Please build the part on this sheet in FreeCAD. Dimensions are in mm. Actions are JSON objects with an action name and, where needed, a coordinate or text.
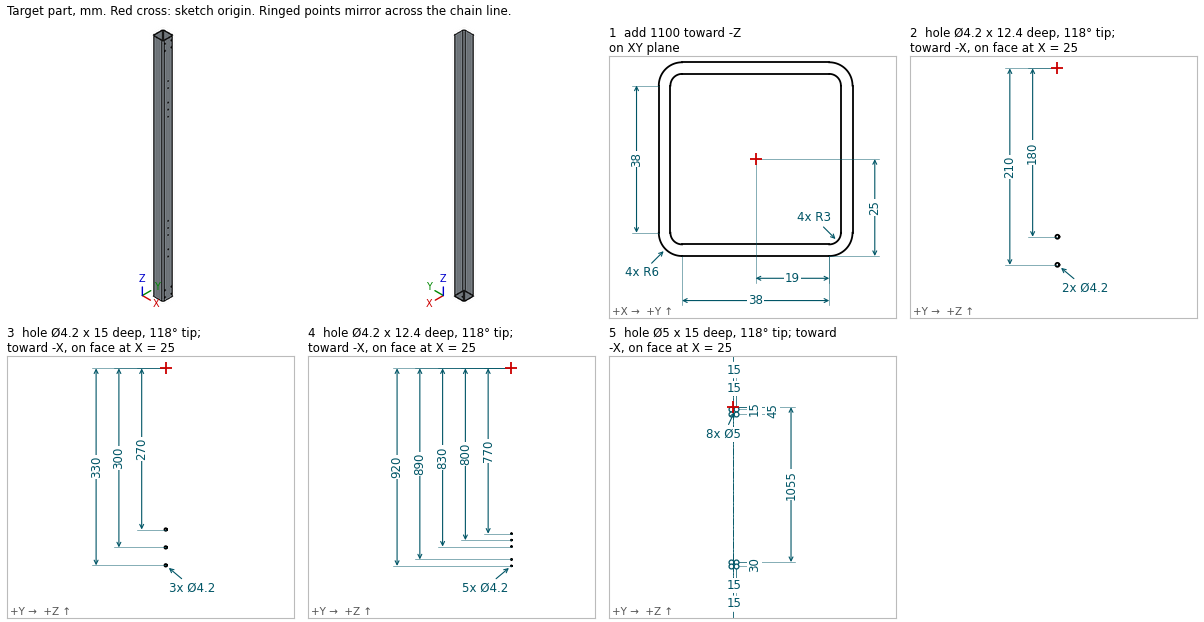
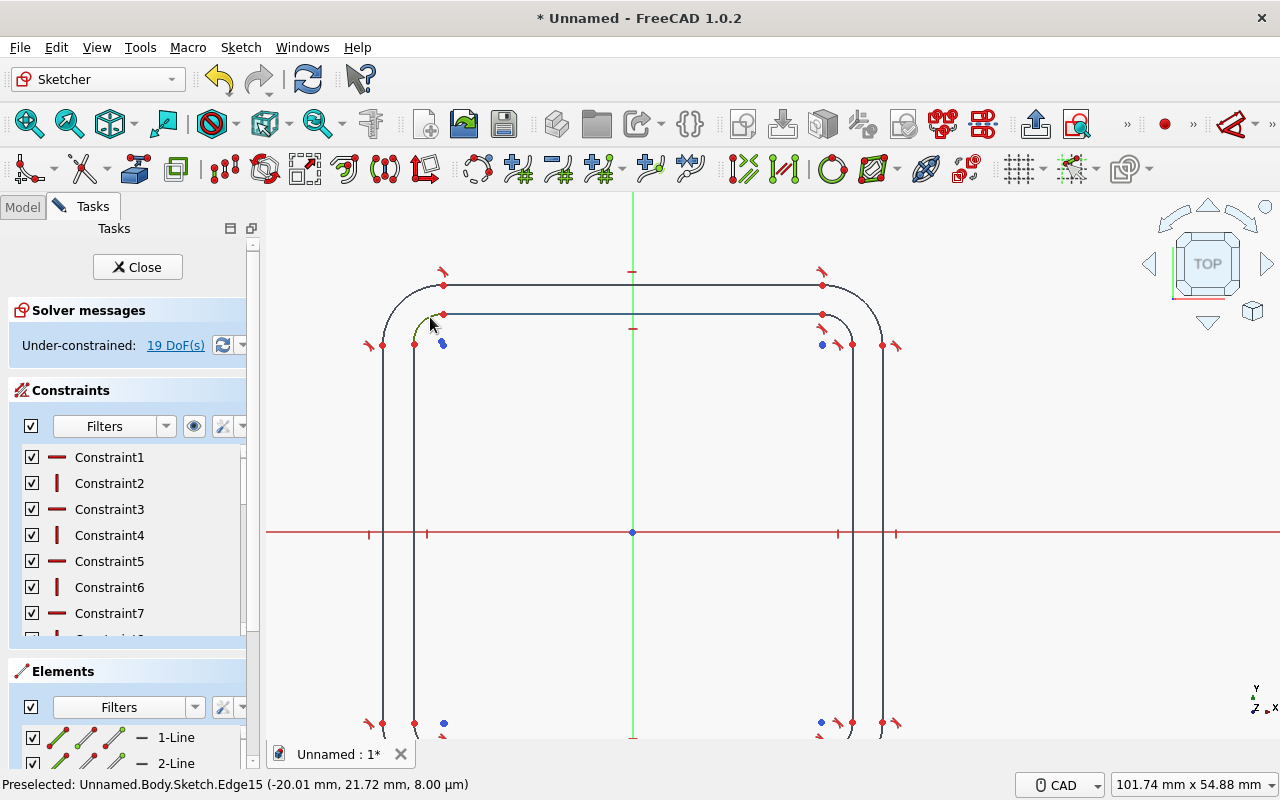
{"action": "key", "text": "t"}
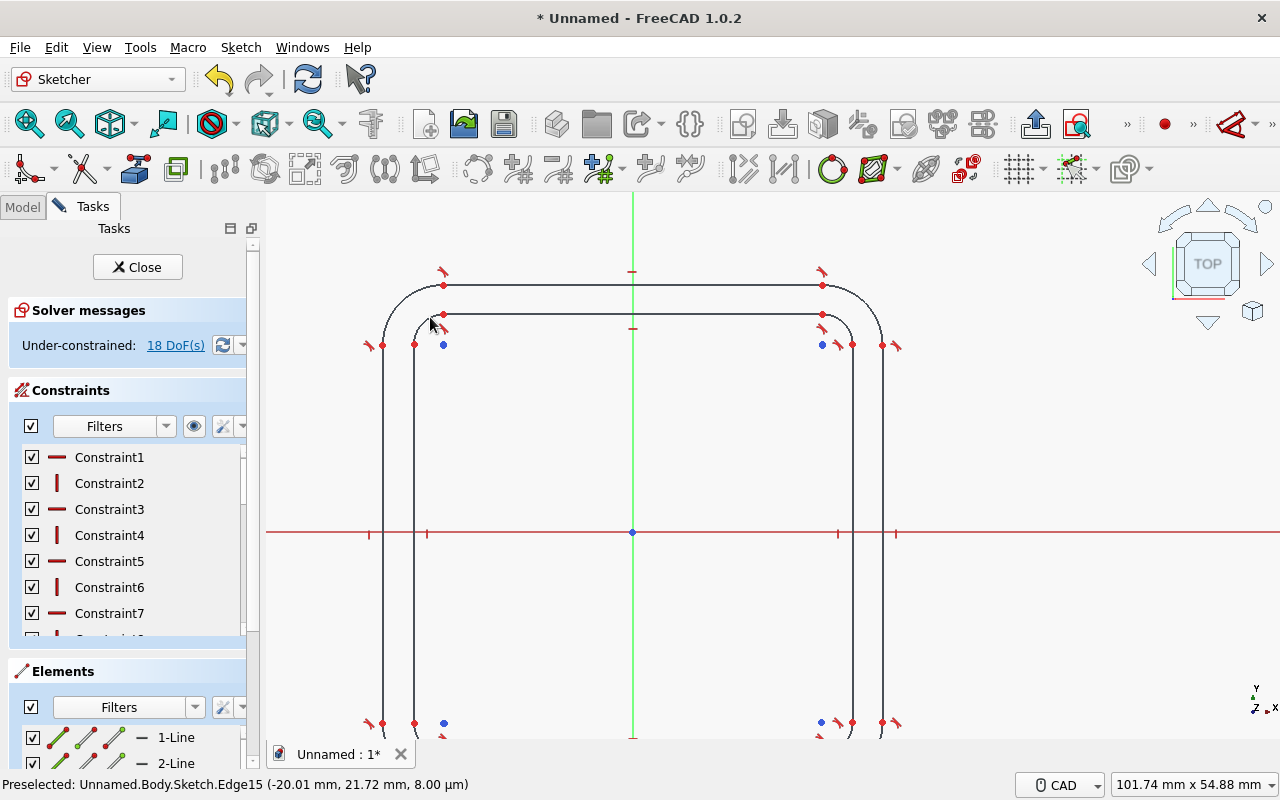
{"action": "left_click", "coordinate": [414, 458]}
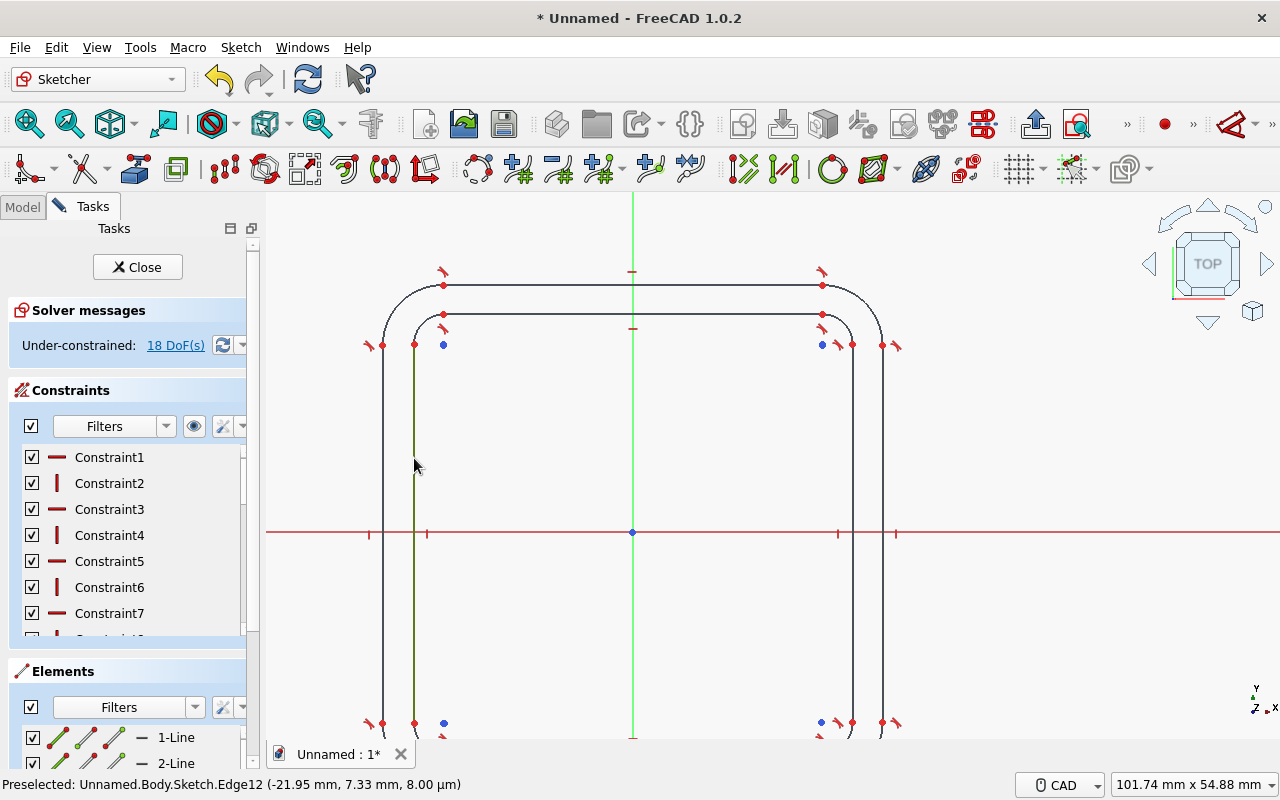
{"action": "left_click", "coordinate": [430, 318]}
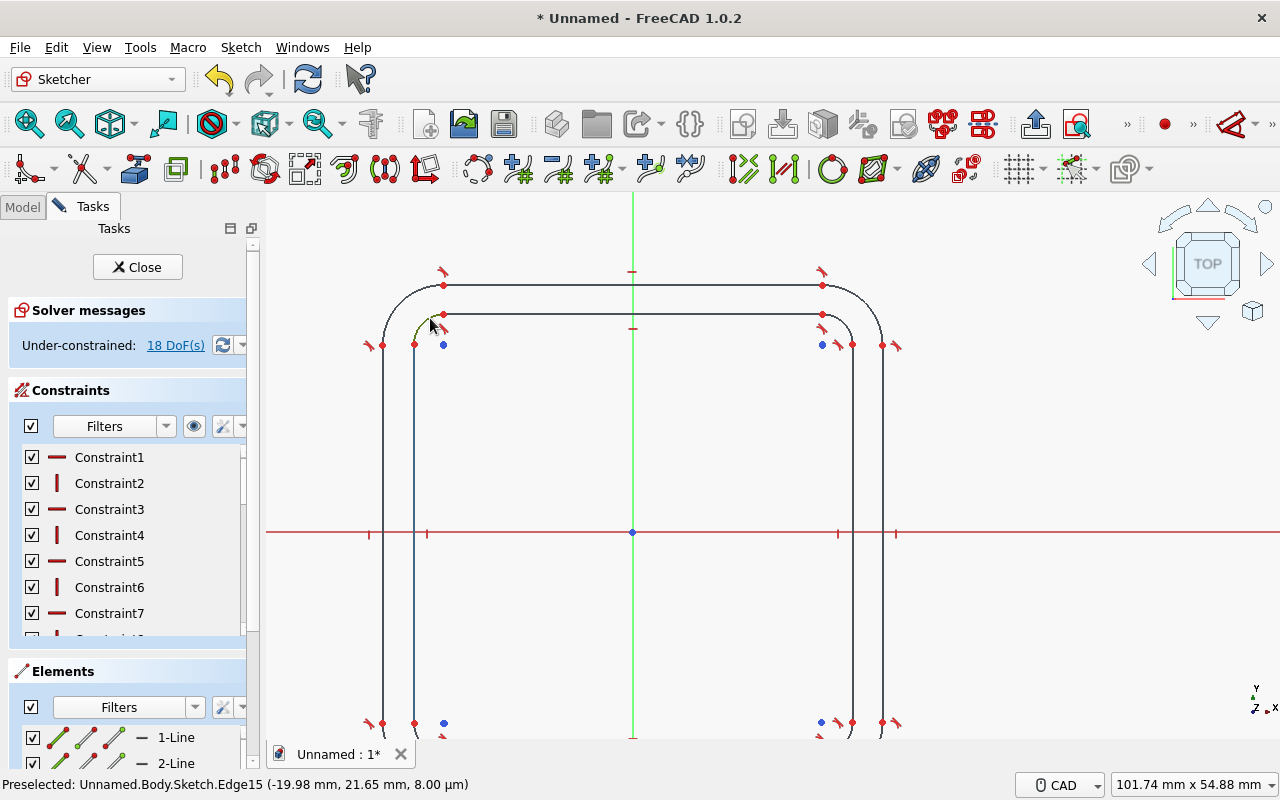
{"action": "key", "text": "t"}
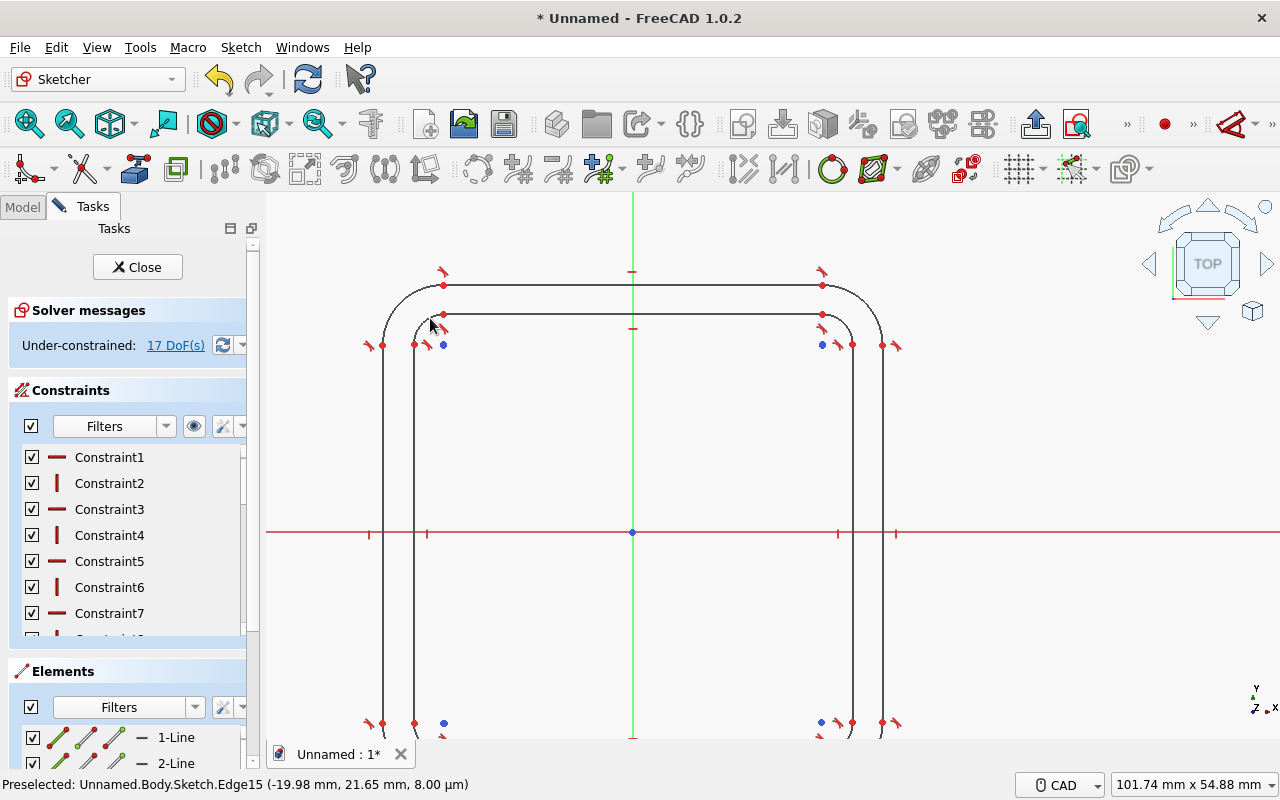
{"action": "left_click", "coordinate": [414, 458]}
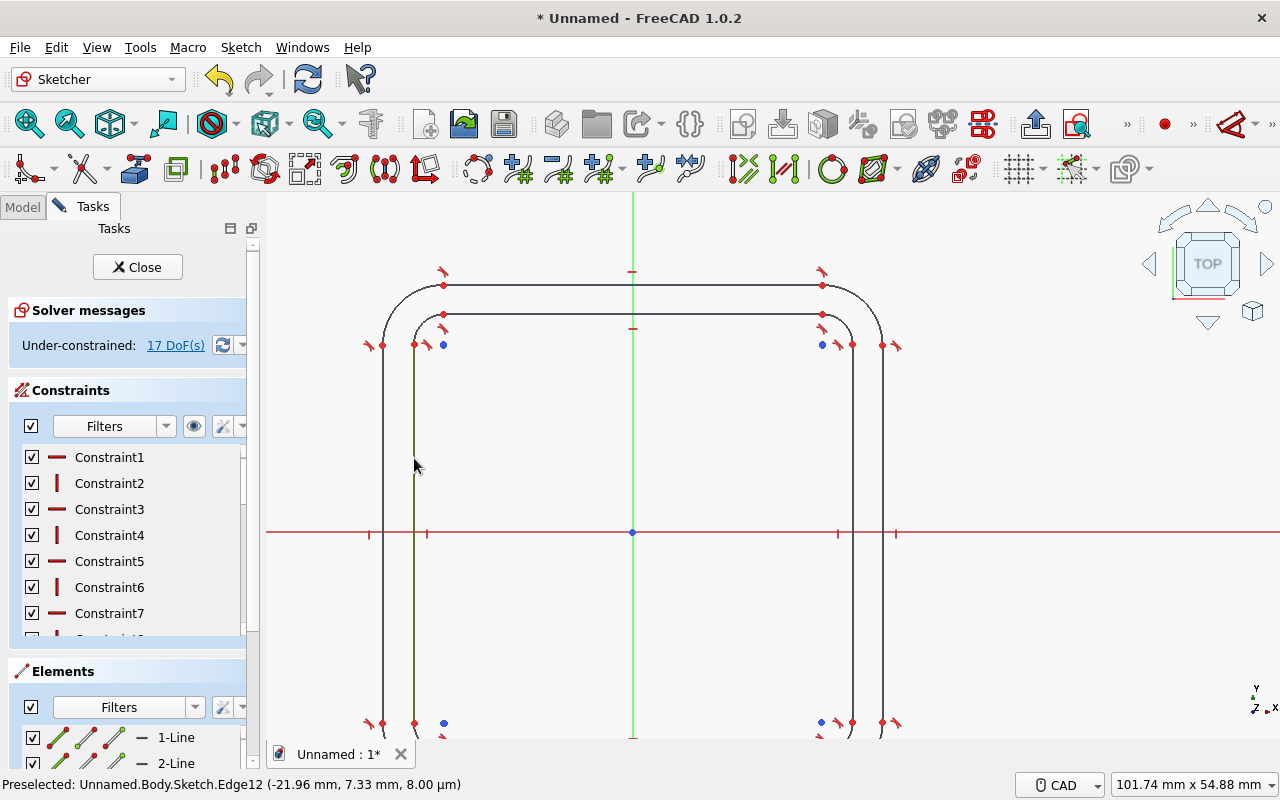
{"action": "scroll", "coordinate": [850, 330], "scroll_direction": "down", "scroll_amount": 2}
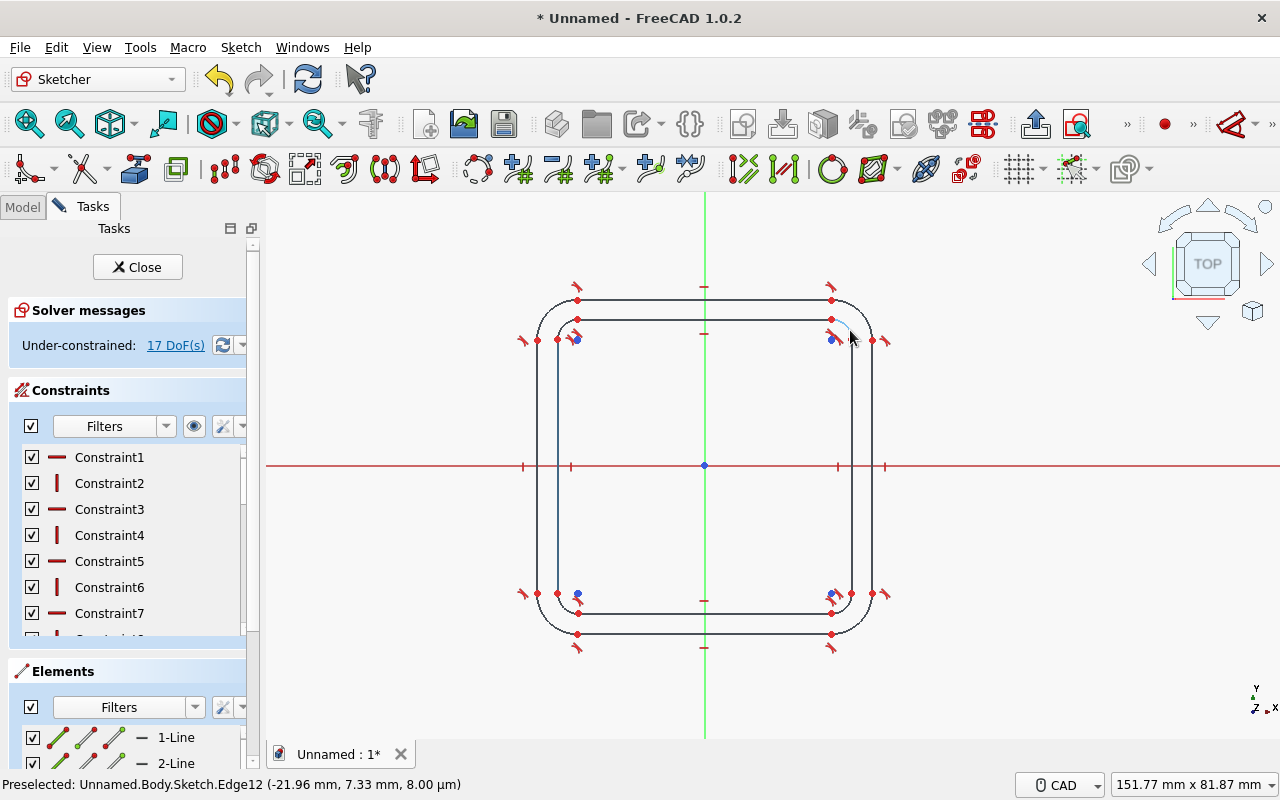
{"action": "scroll", "coordinate": [560, 603], "scroll_direction": "up", "scroll_amount": 2}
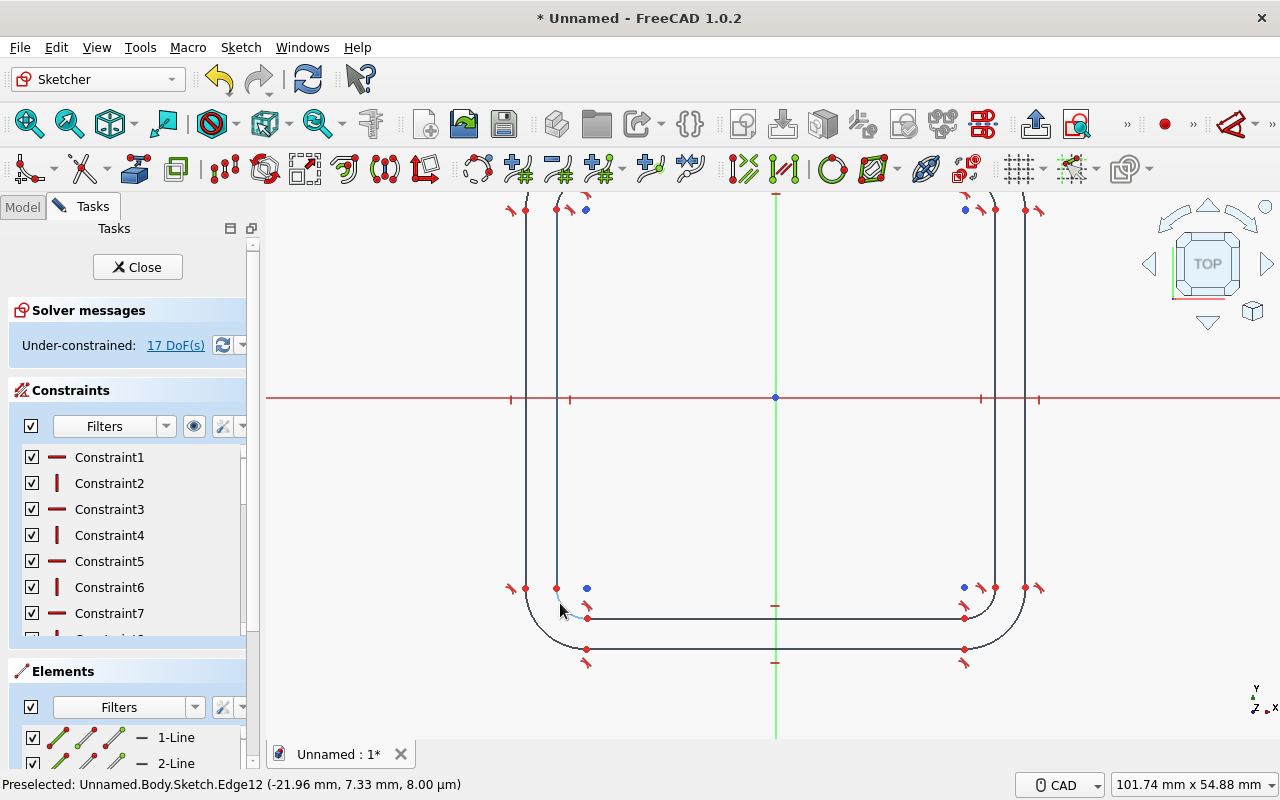
{"action": "left_click", "coordinate": [560, 602]}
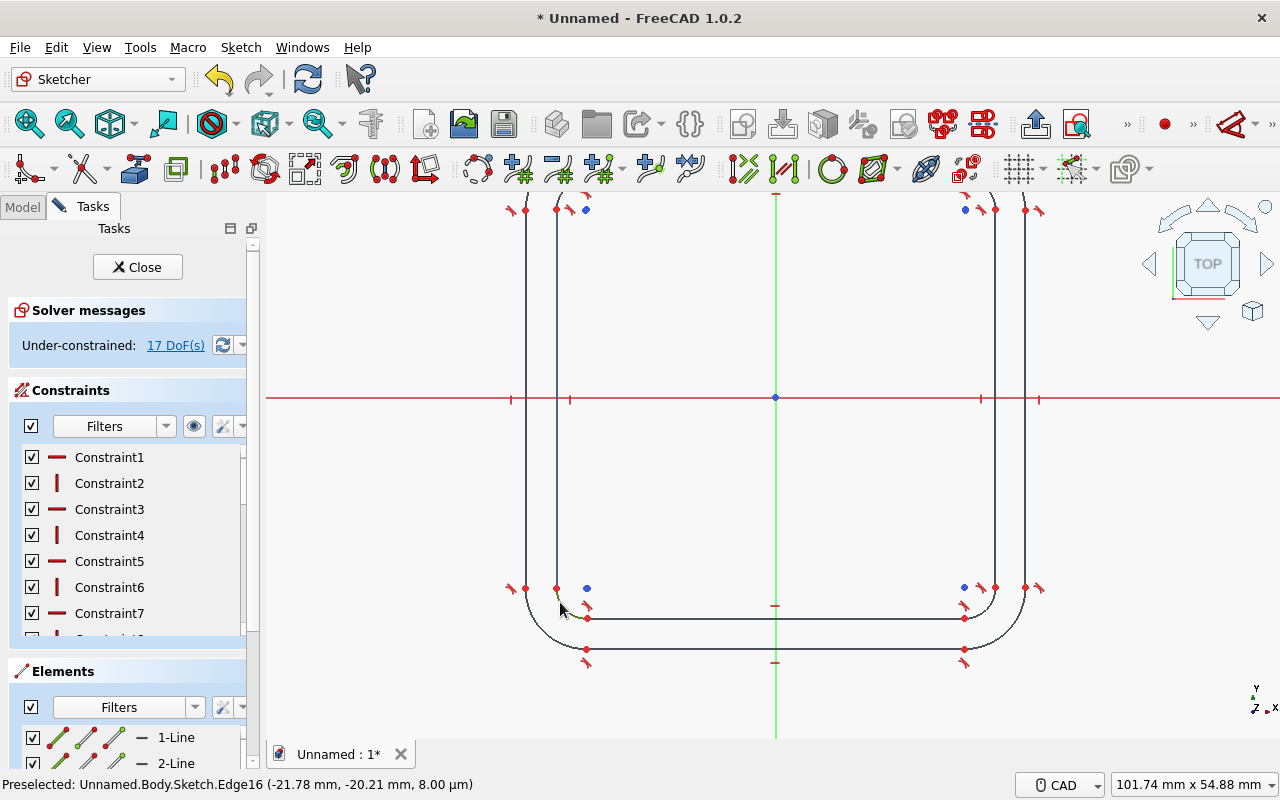
{"action": "key", "text": "t"}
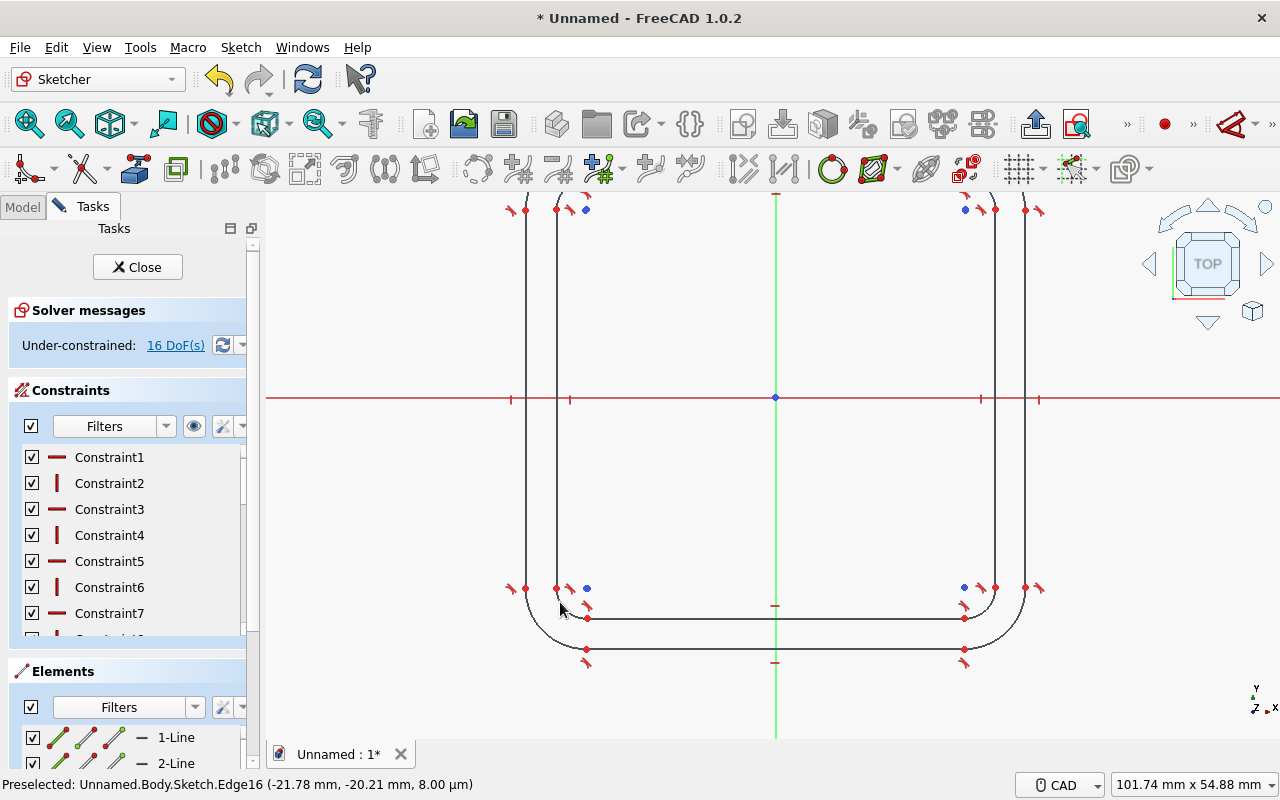
{"action": "left_click", "coordinate": [992, 642]}